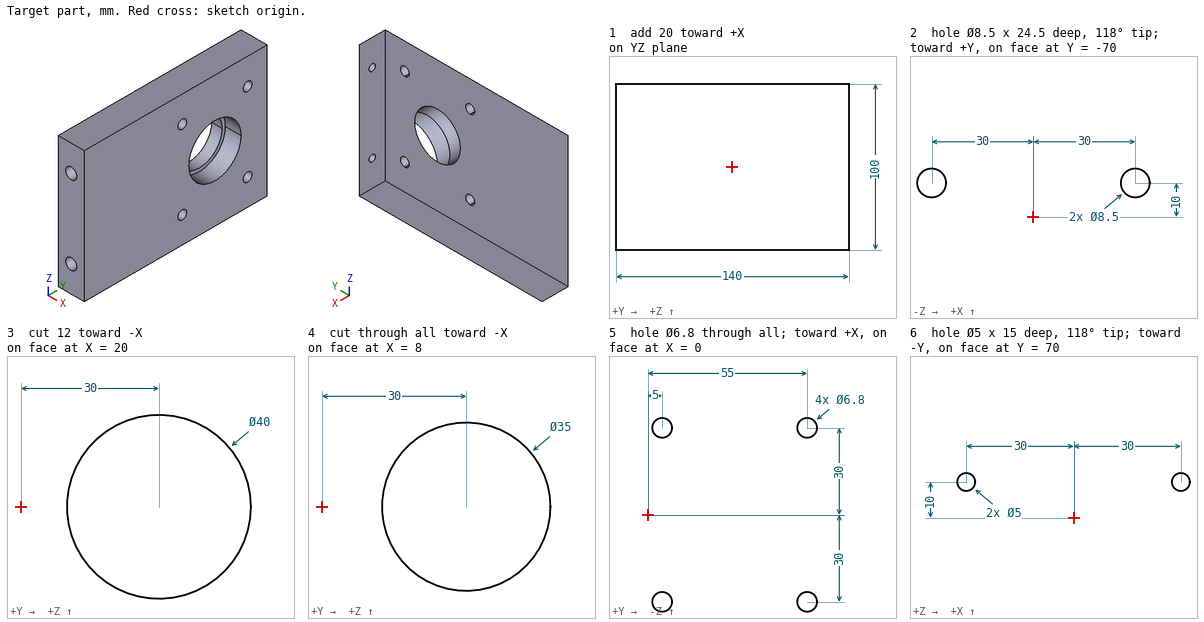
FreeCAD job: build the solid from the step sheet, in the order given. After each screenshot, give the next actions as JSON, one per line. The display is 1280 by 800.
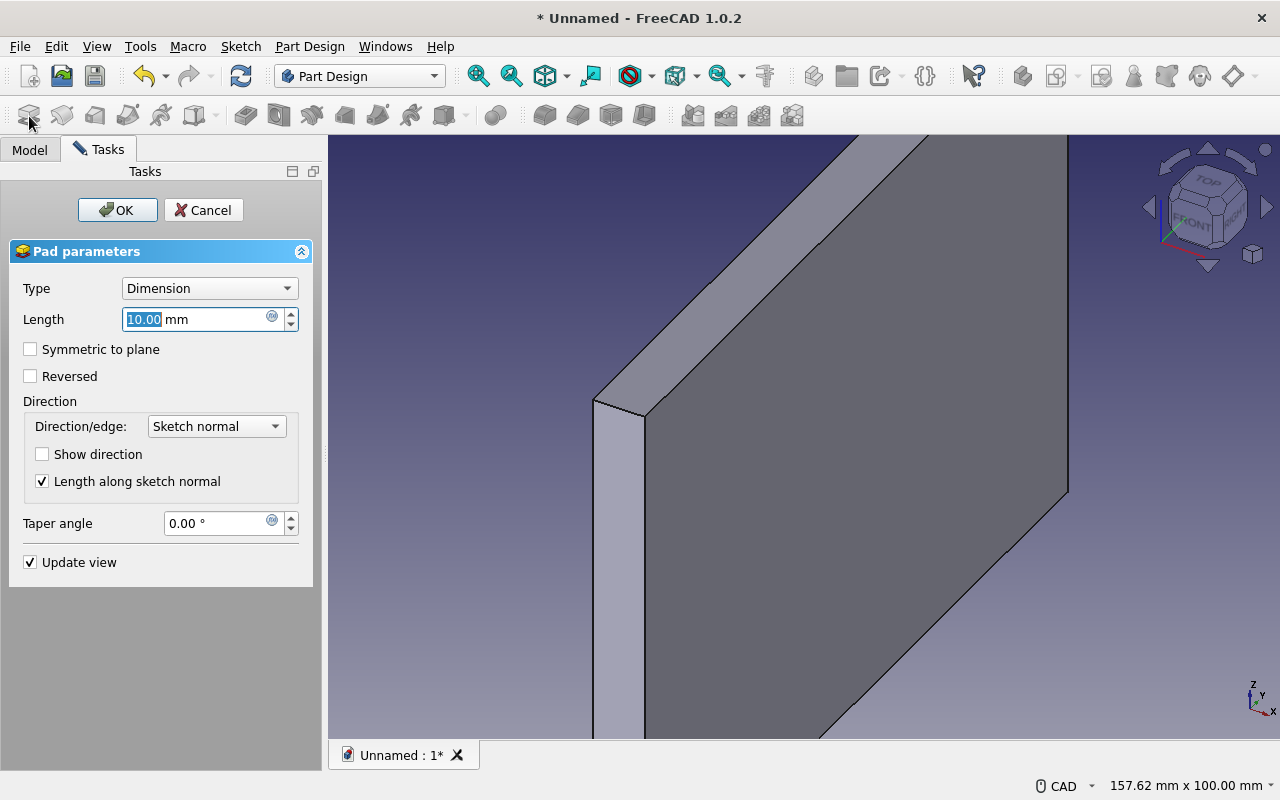
{"action": "type", "text": "20"}
{"action": "key", "text": "Tab"}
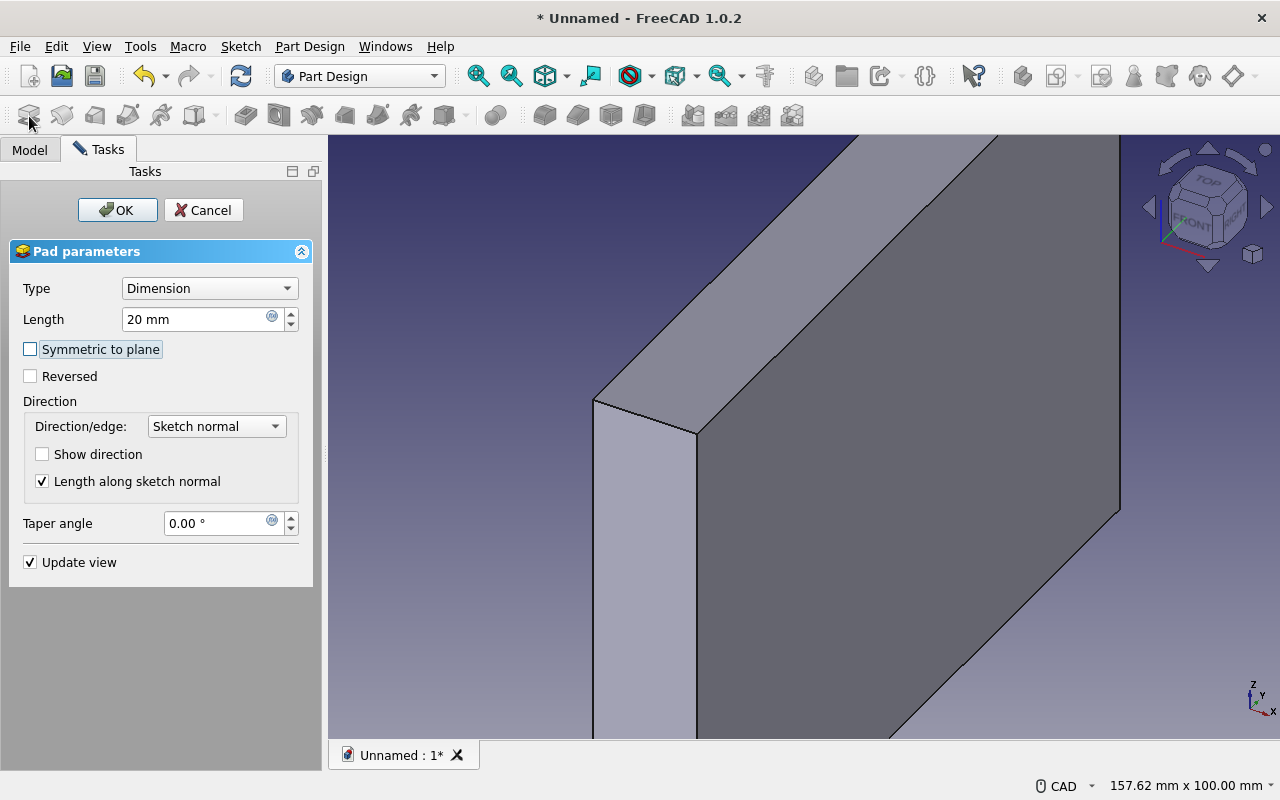
{"action": "left_click", "coordinate": [118, 210]}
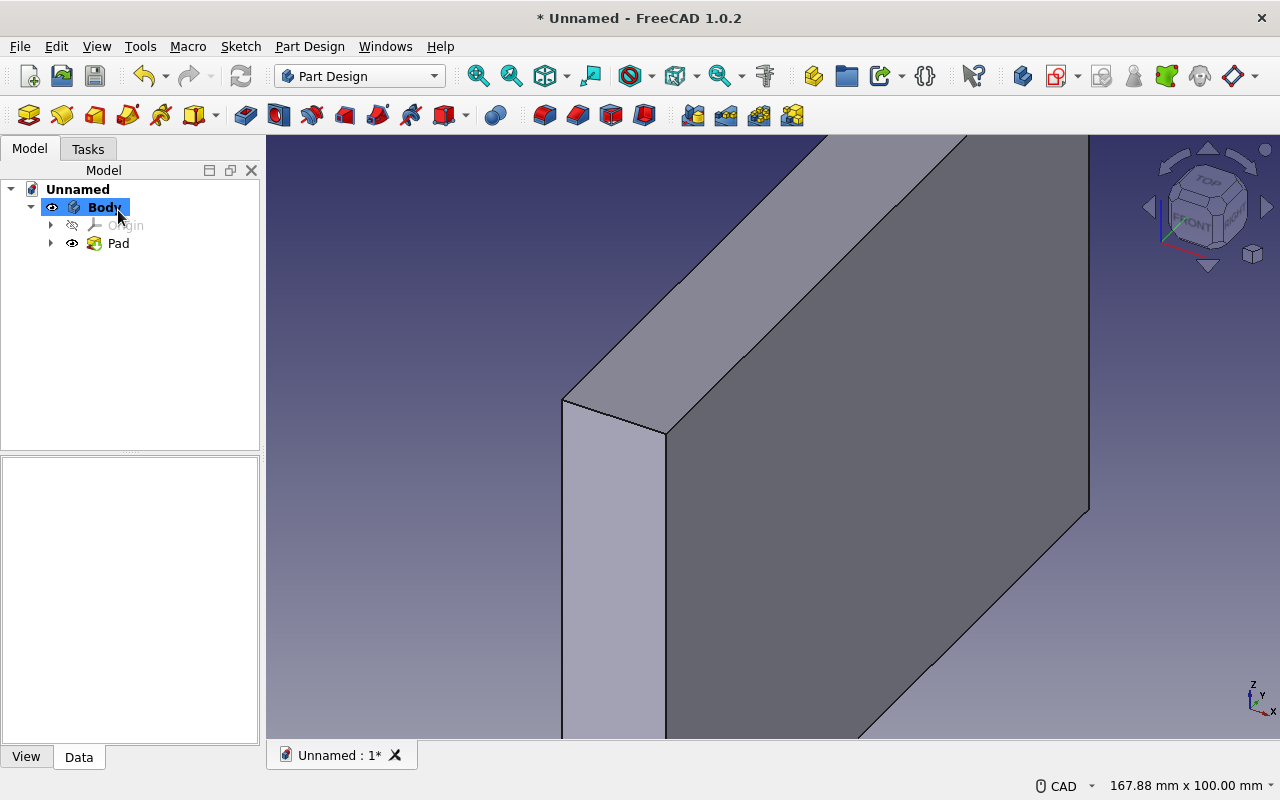
{"action": "left_click", "coordinate": [479, 76]}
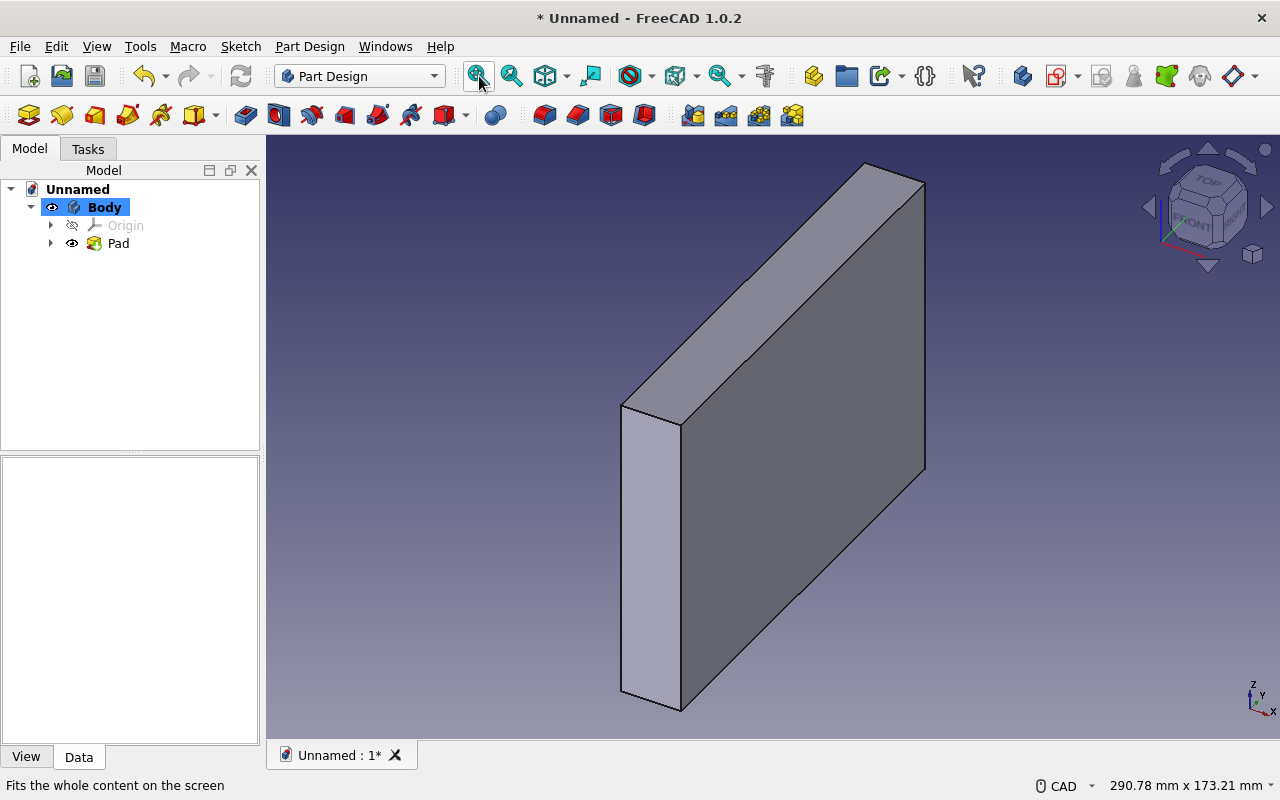
{"action": "left_click", "coordinate": [651, 557]}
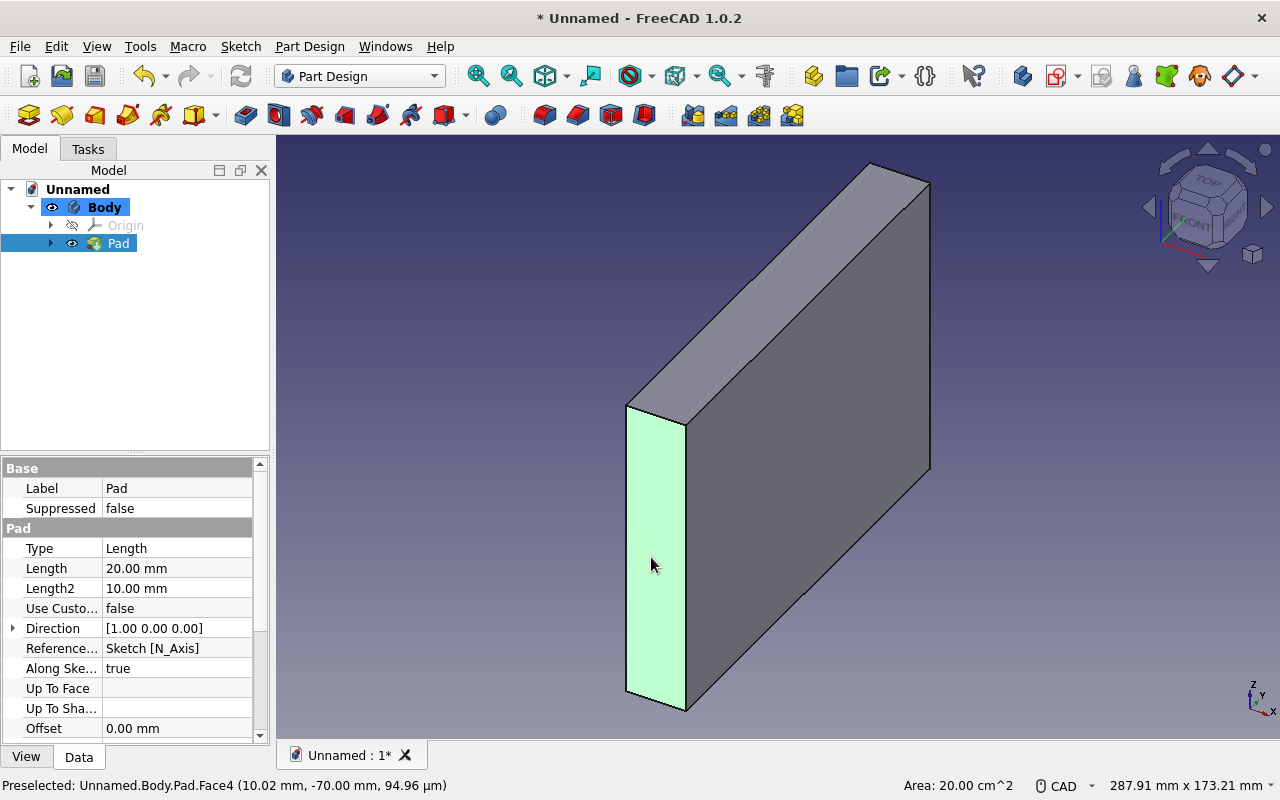
{"action": "left_click", "coordinate": [1056, 76]}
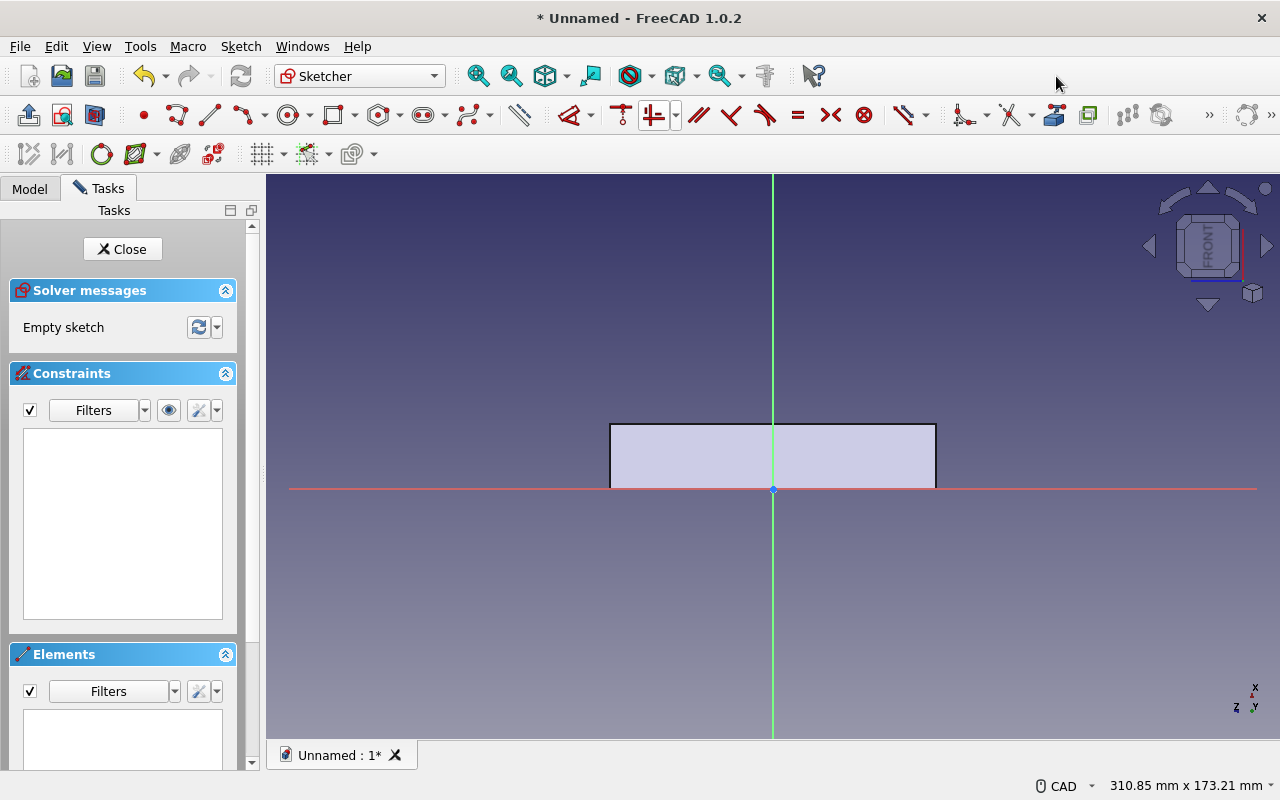
{"action": "scroll", "coordinate": [813, 471], "scroll_direction": "up", "scroll_amount": 5}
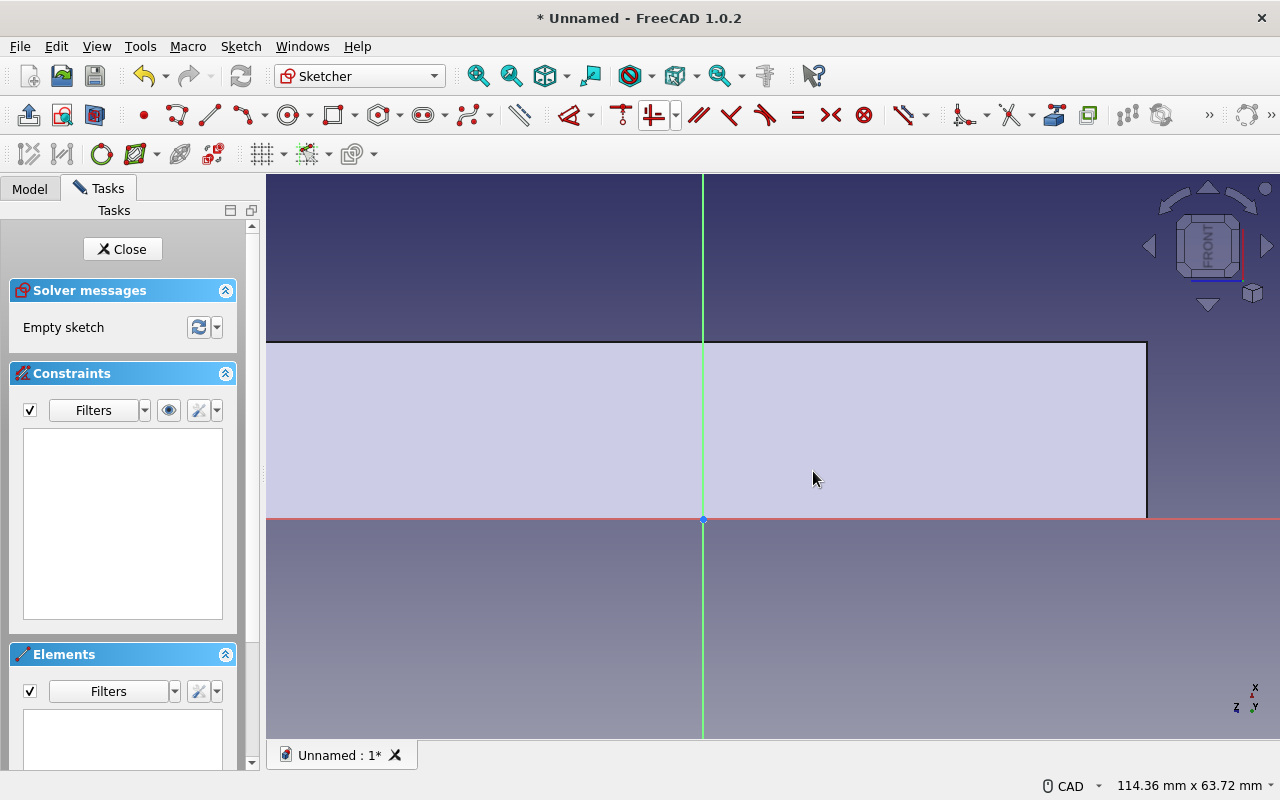
{"action": "key", "text": "g c"}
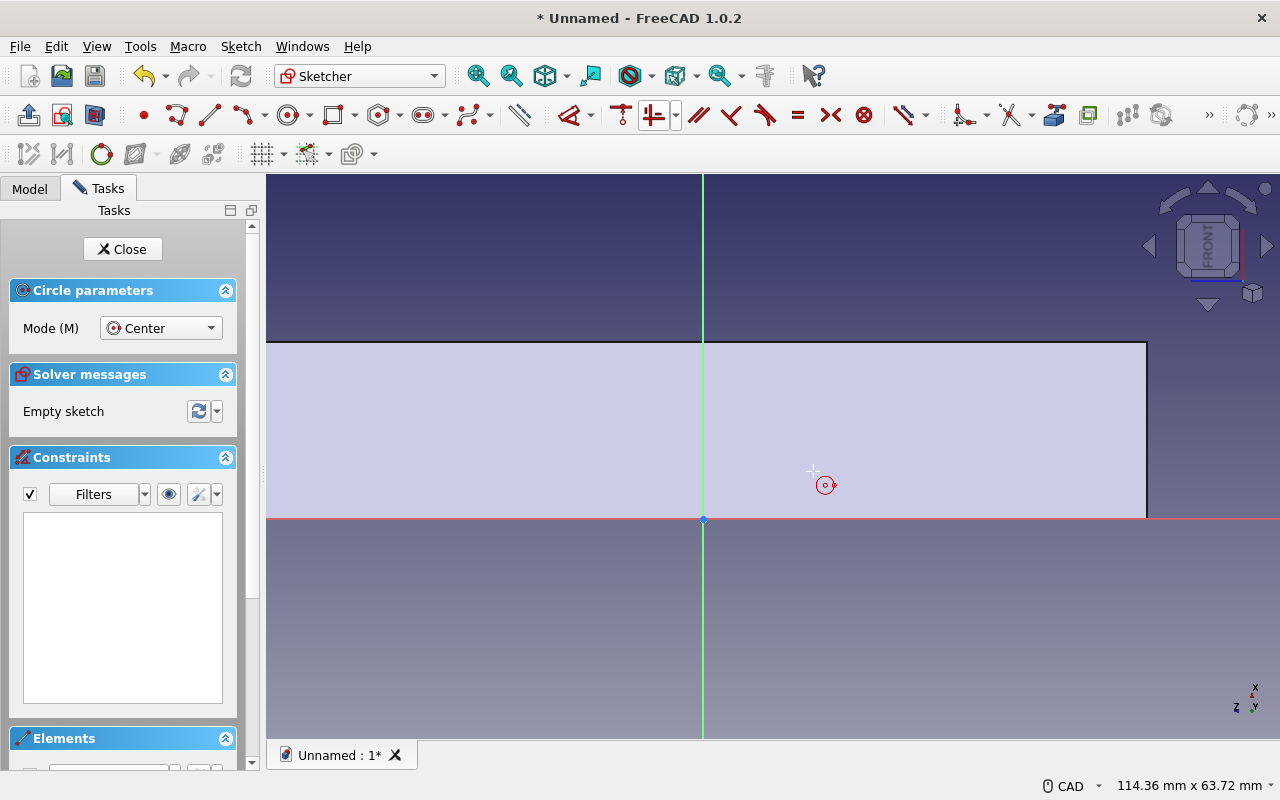
{"action": "left_click", "coordinate": [969, 431]}
{"action": "mouse_move", "coordinate": [996, 404]}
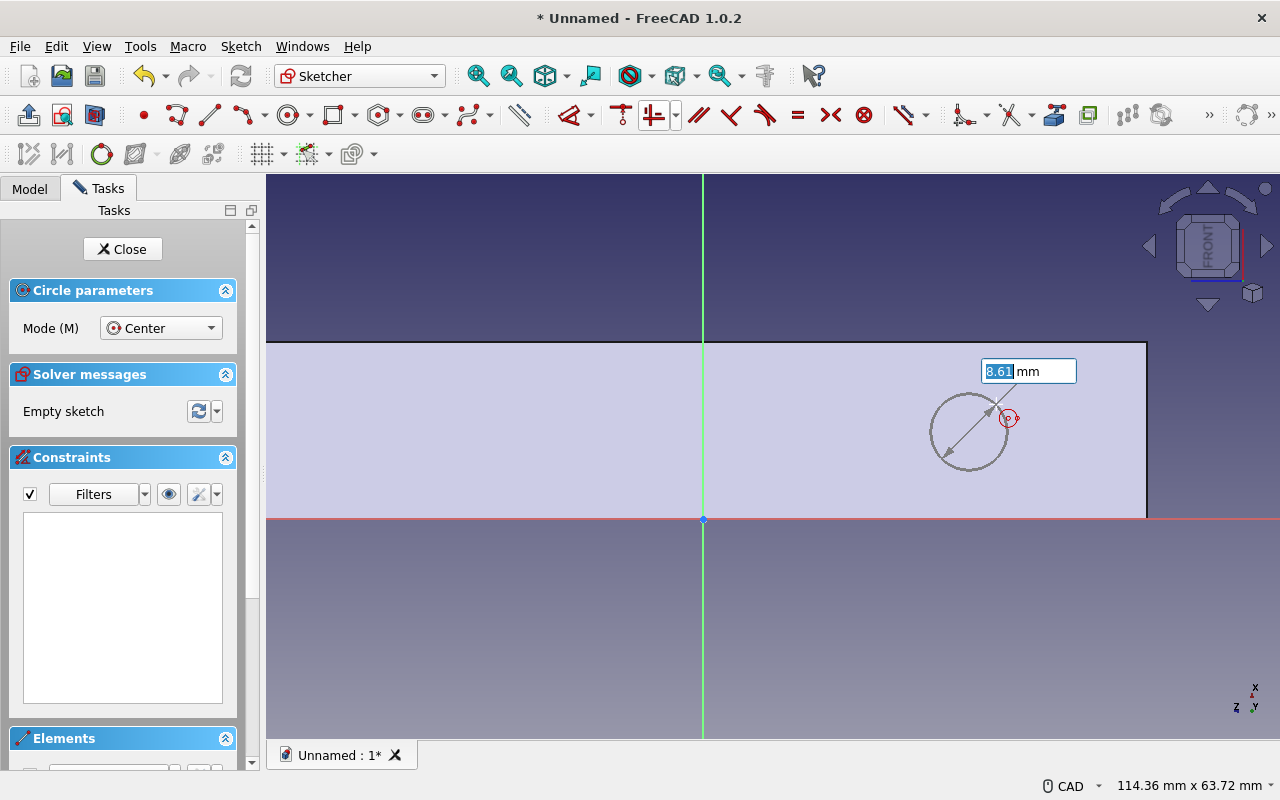
{"action": "type", "text": "8.5"}
{"action": "key", "text": "Return"}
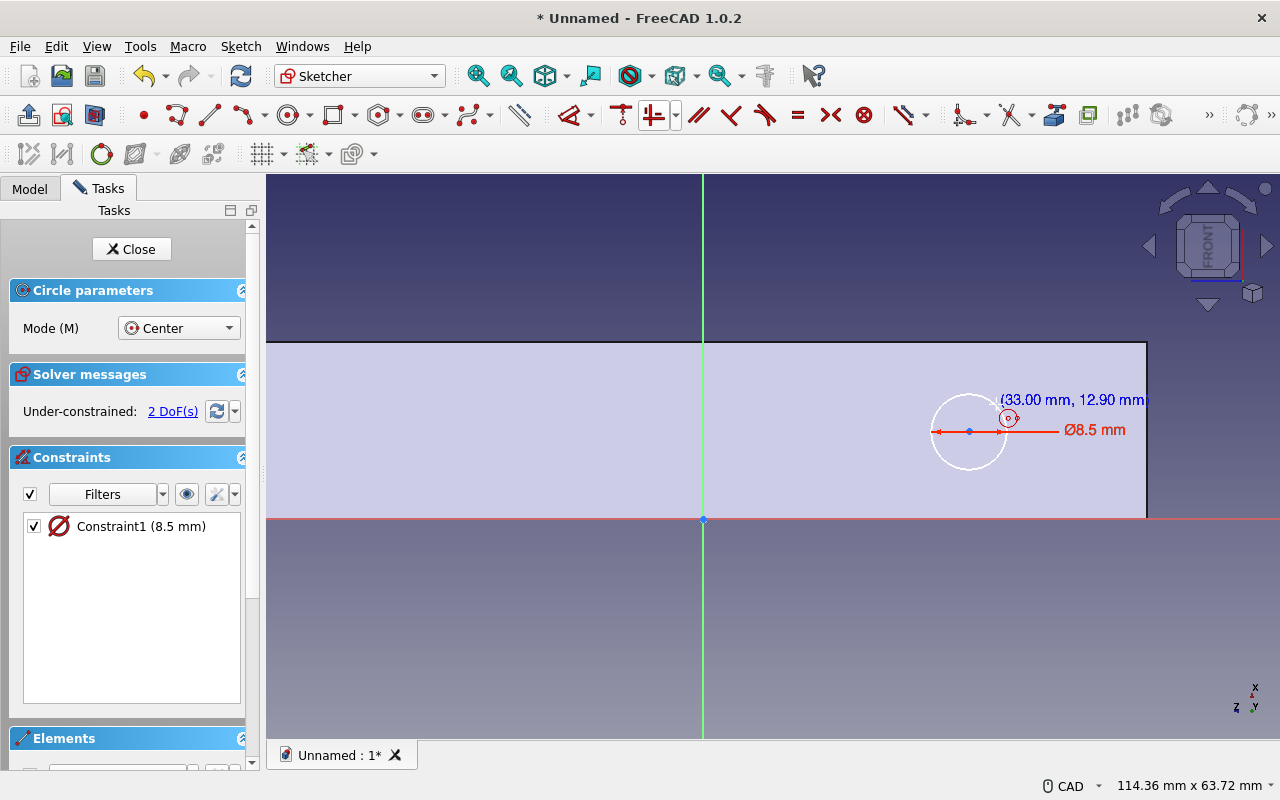
{"action": "left_click", "coordinate": [437, 431]}
{"action": "mouse_move", "coordinate": [464, 404]}